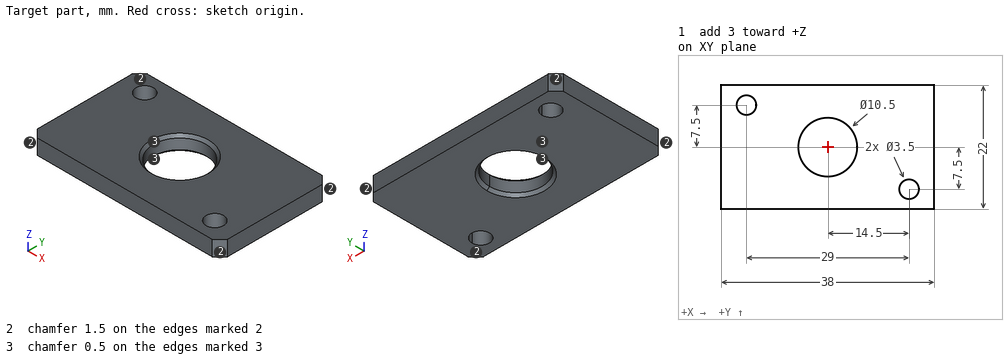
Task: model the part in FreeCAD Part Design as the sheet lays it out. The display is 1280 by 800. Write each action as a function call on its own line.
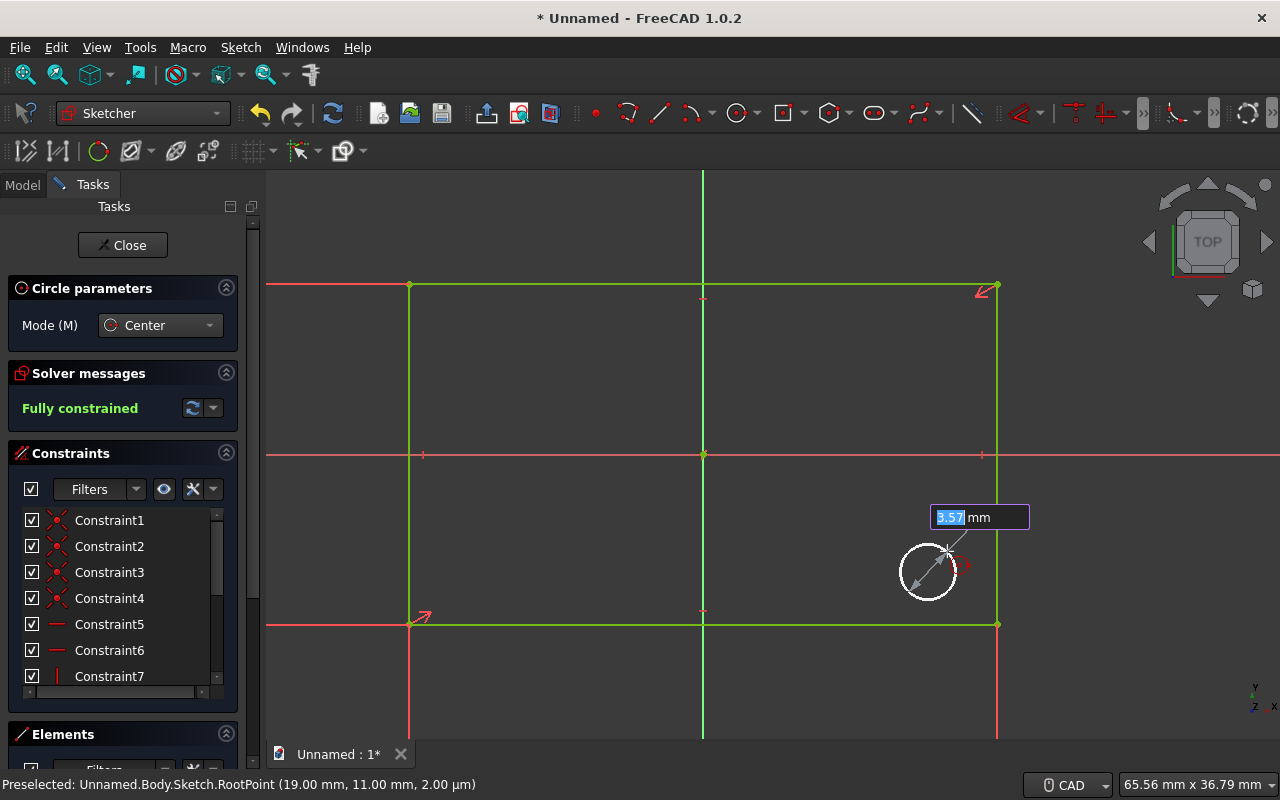
text(3.5)
key(Return)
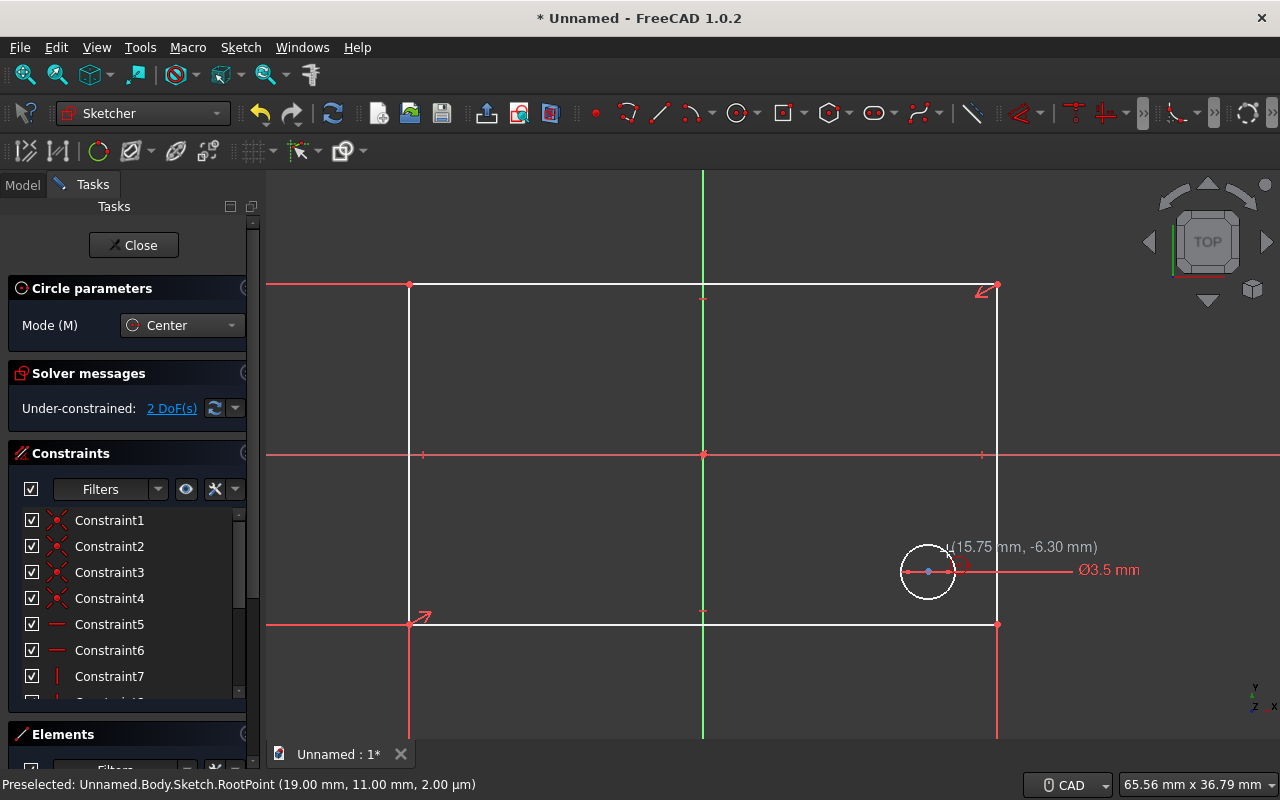
click(479, 338)
move(498, 319)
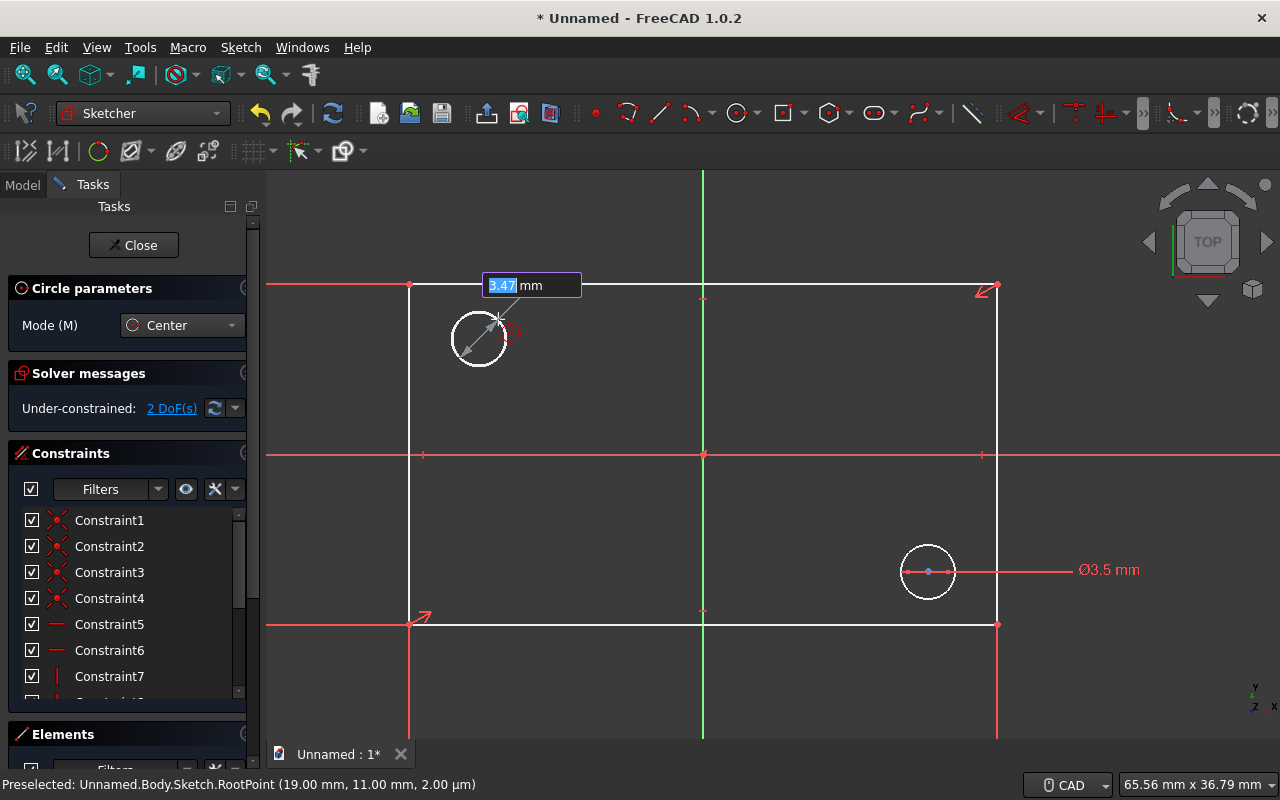
text(3.5)
key(Return)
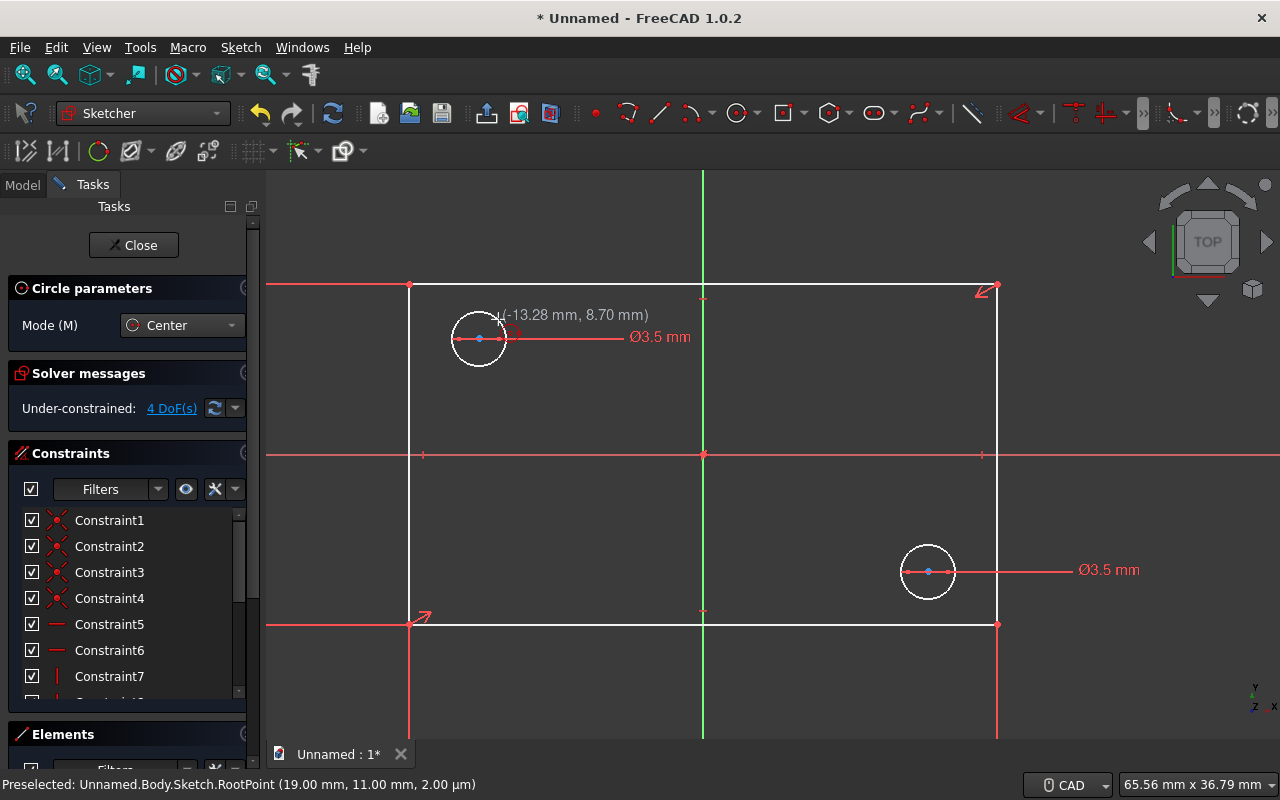
click(703, 454)
move(761, 397)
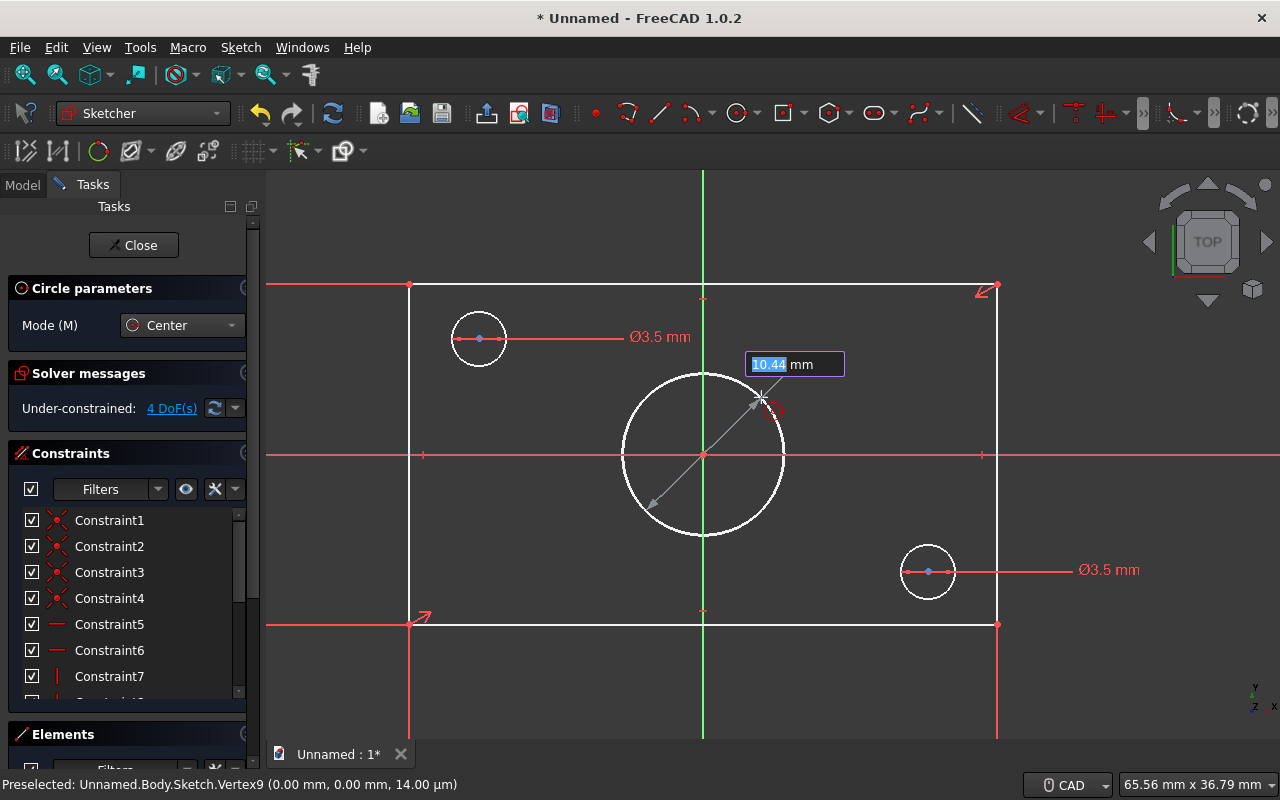
text(10.5)
key(Return)
key(Escape)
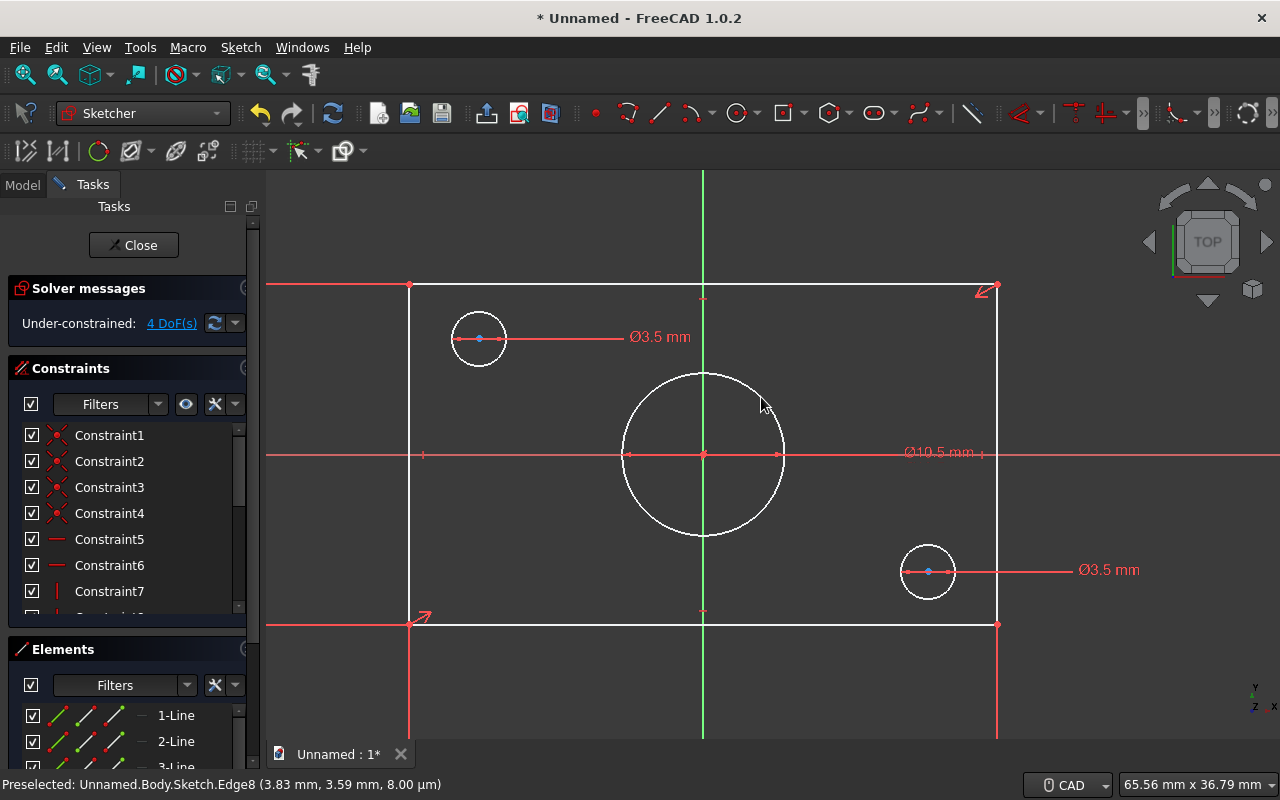
key(d)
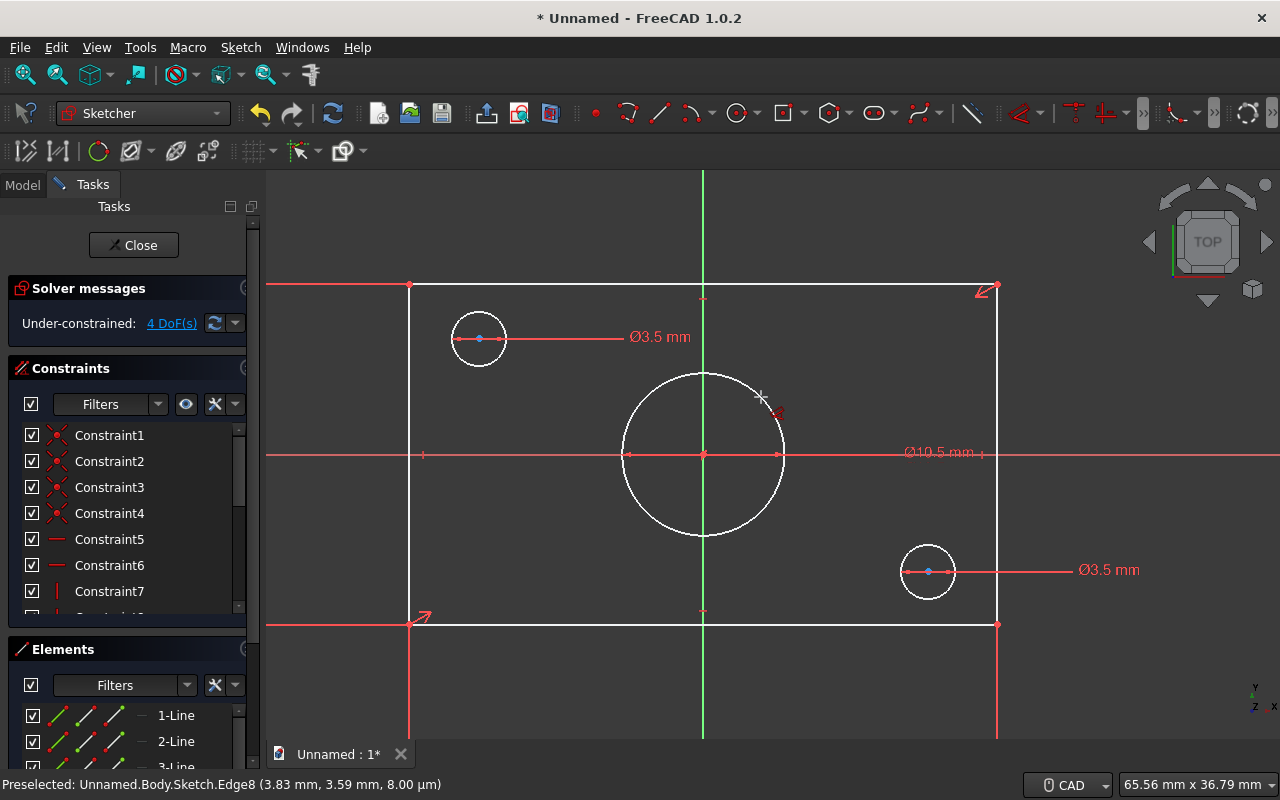
click(928, 572)
click(962, 513)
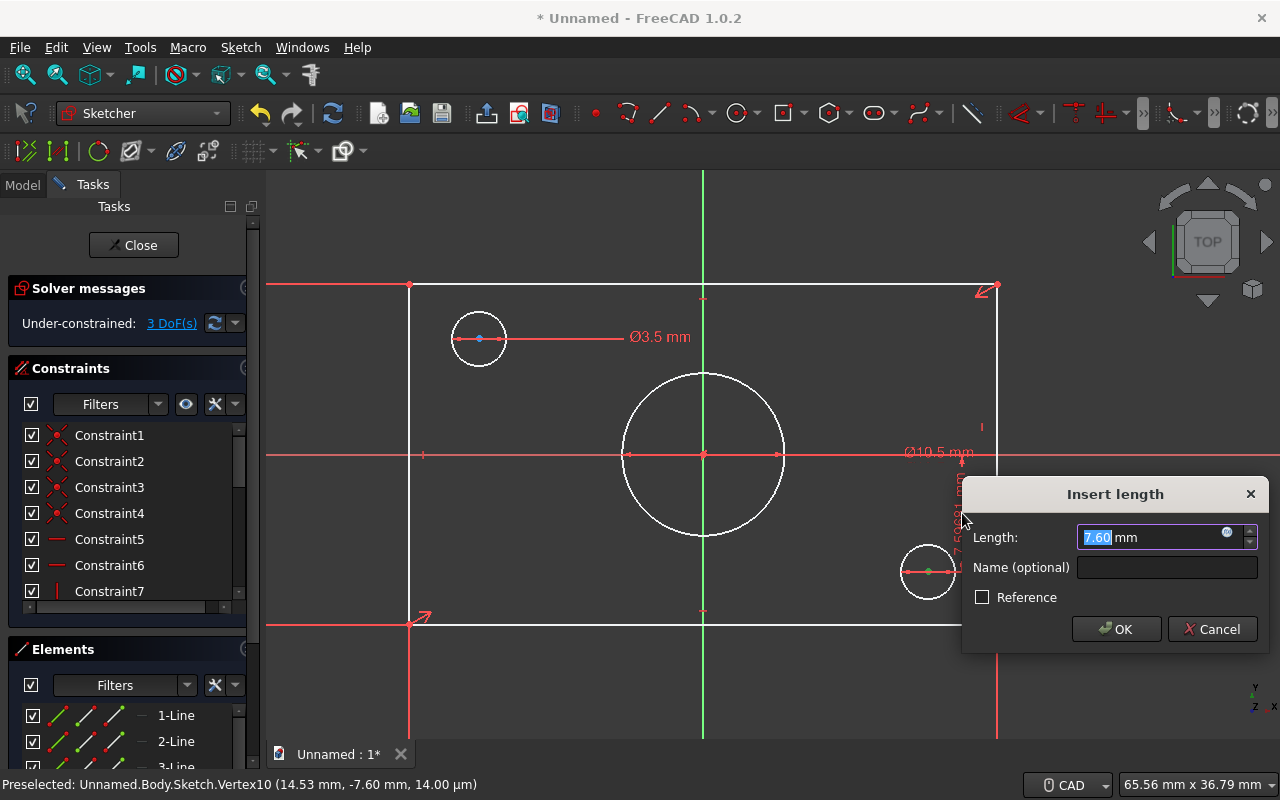
text(7.5)
key(Return)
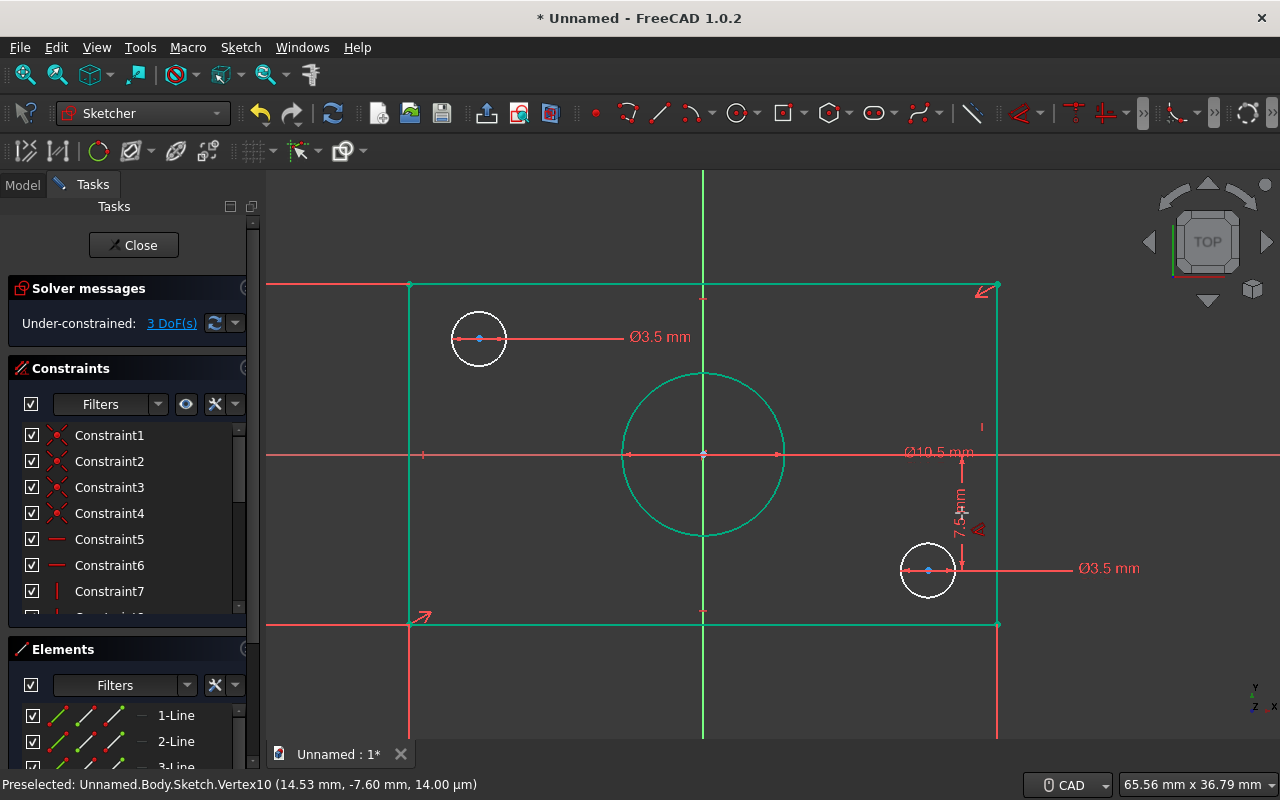
click(479, 339)
click(445, 397)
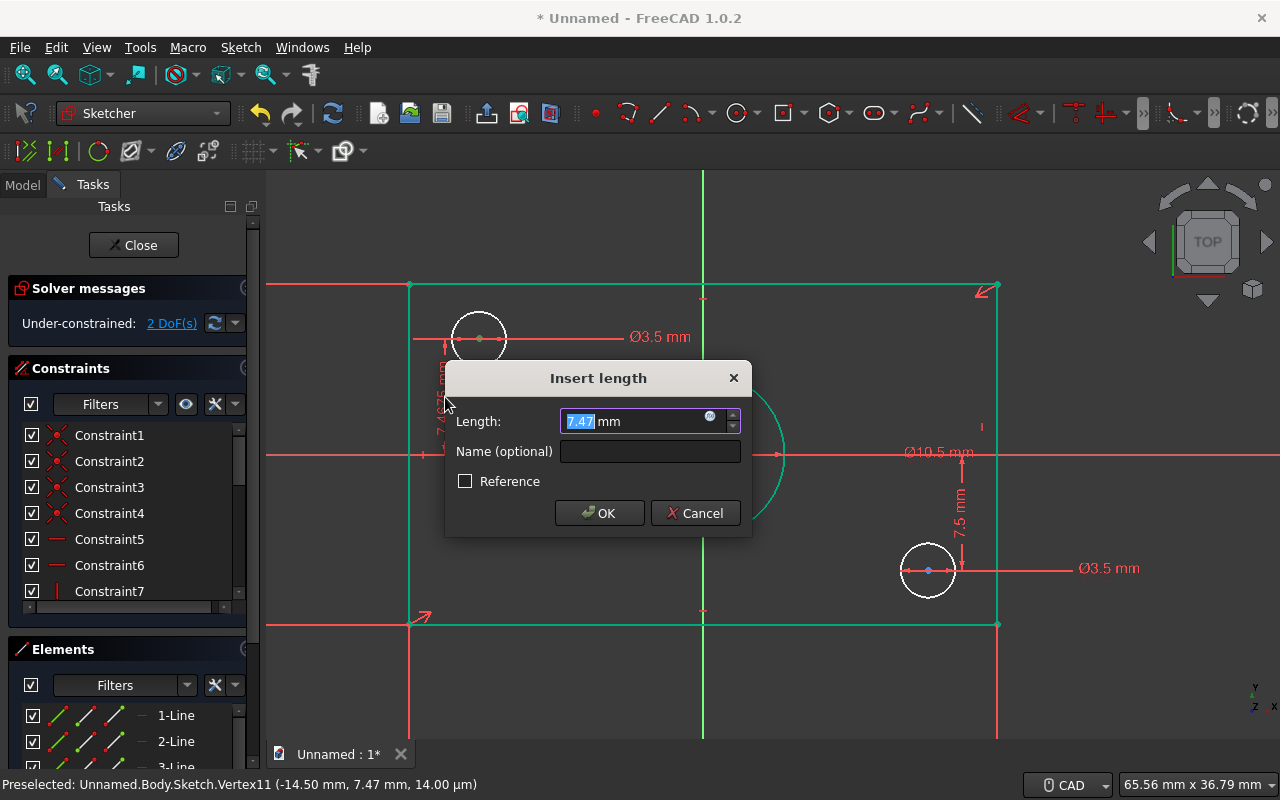
text(7.5)
key(Return)